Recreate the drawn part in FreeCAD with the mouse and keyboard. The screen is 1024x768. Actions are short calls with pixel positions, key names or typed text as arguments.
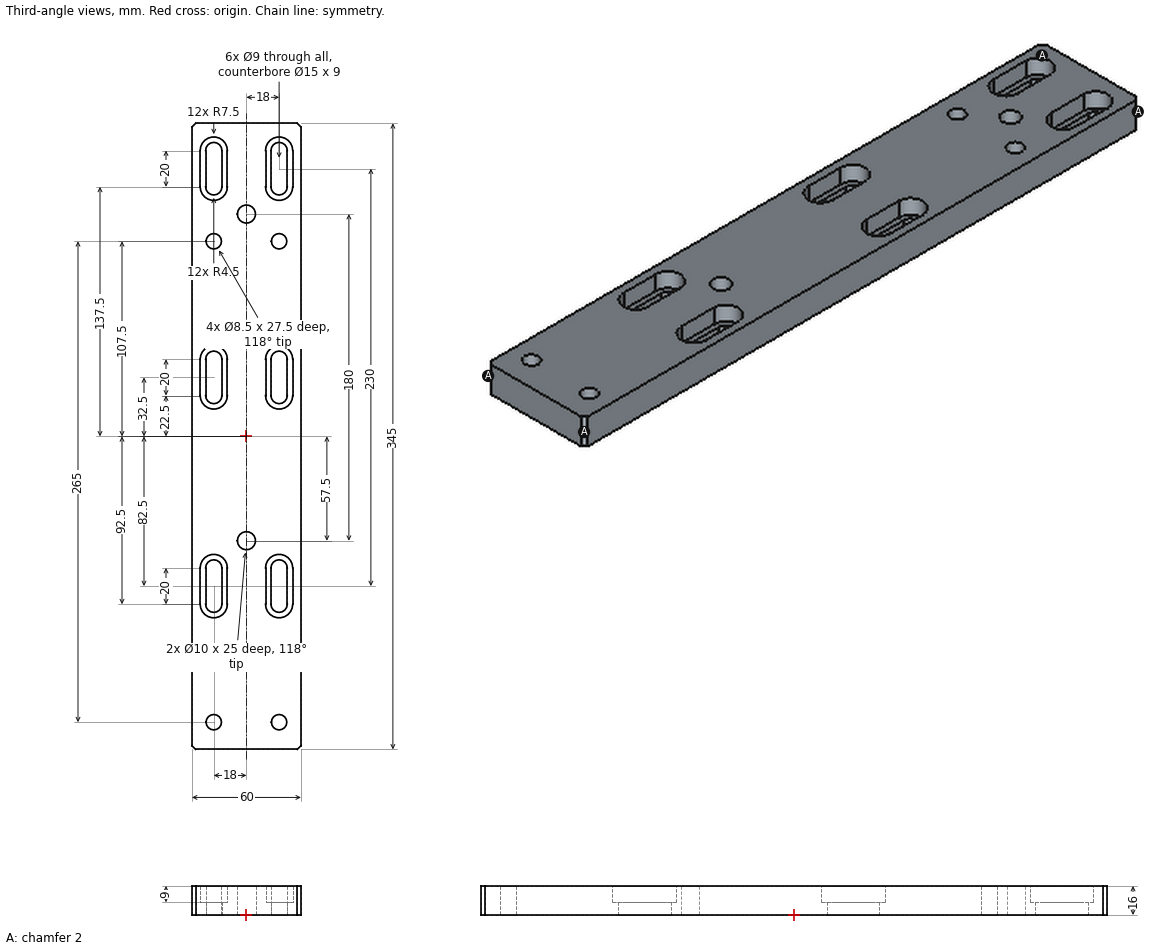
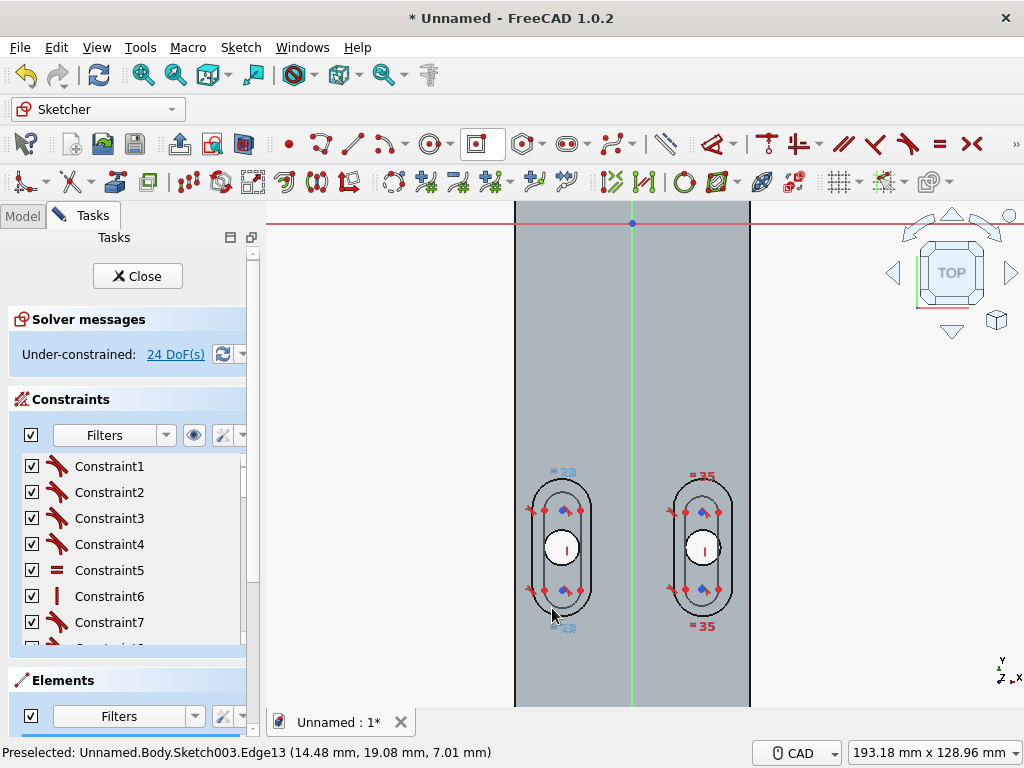
click(552, 605)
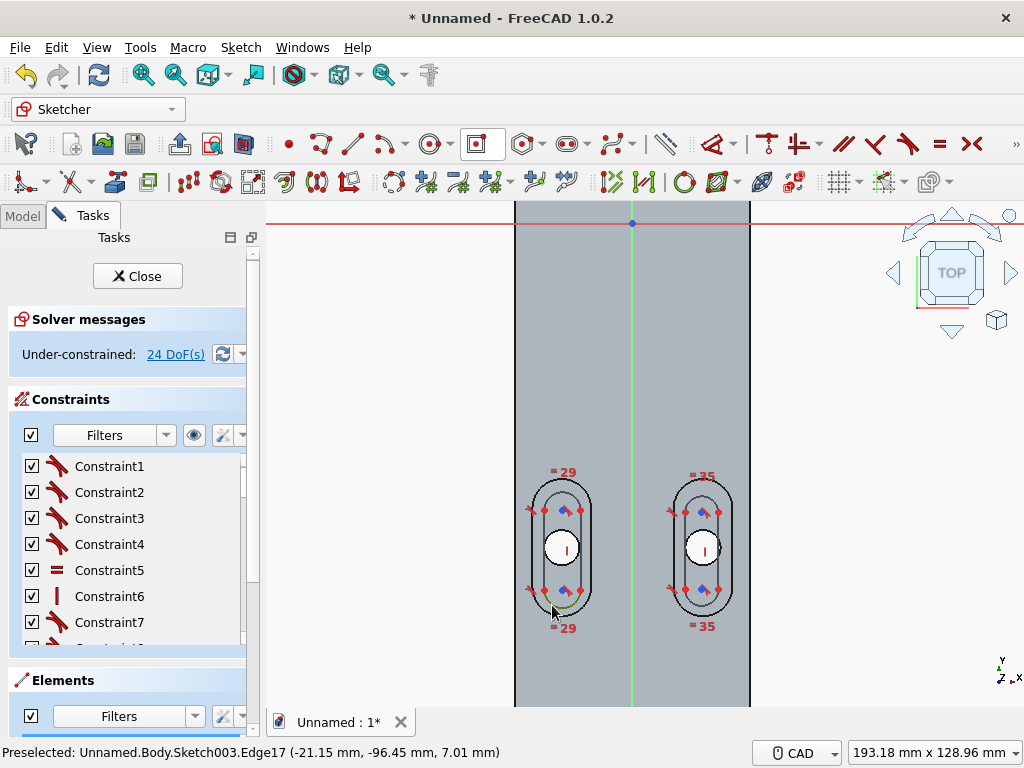
click(692, 603)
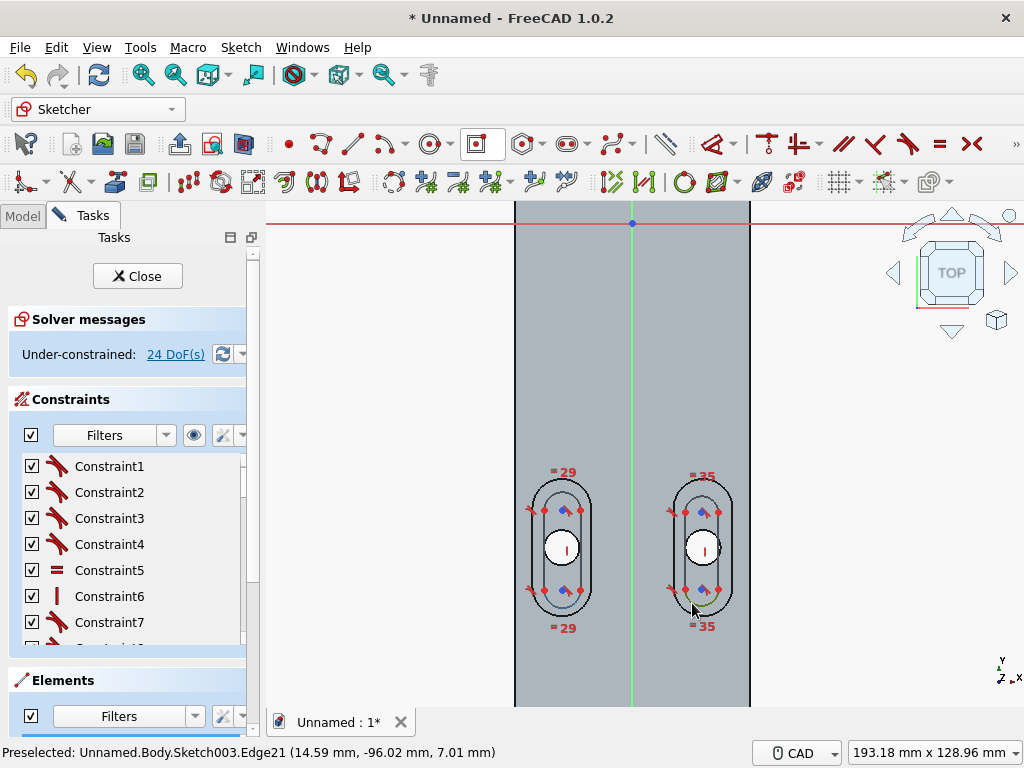
key(e)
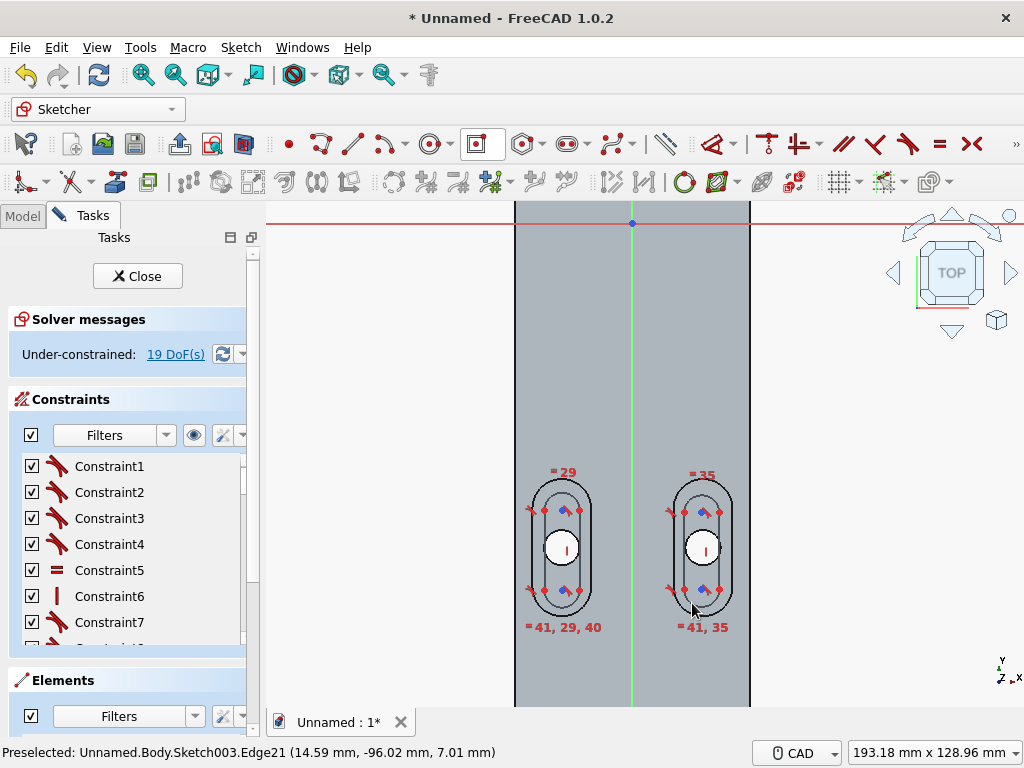
scroll(552, 608, down, 6)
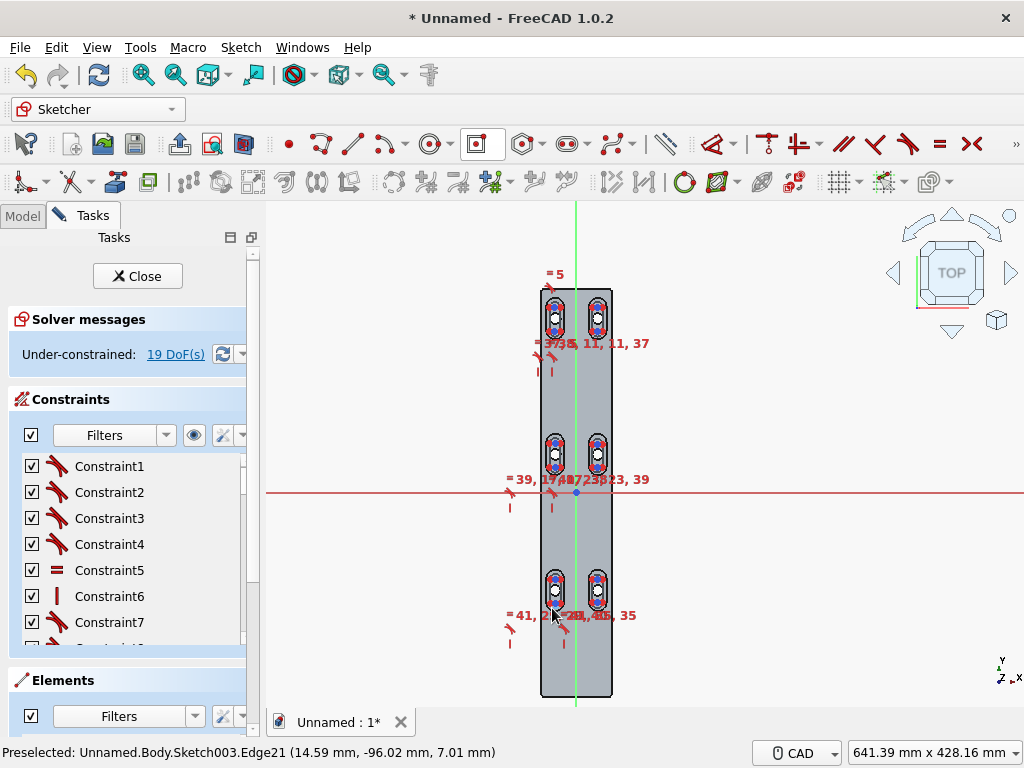
scroll(555, 331, up, 5)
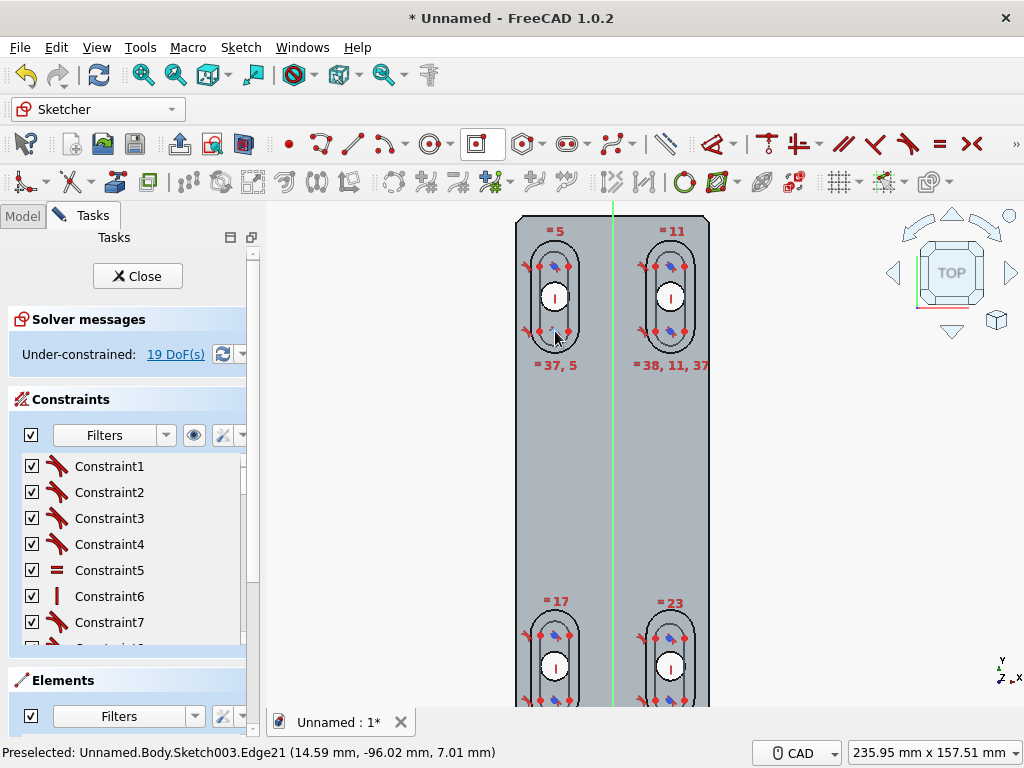
click(554, 331)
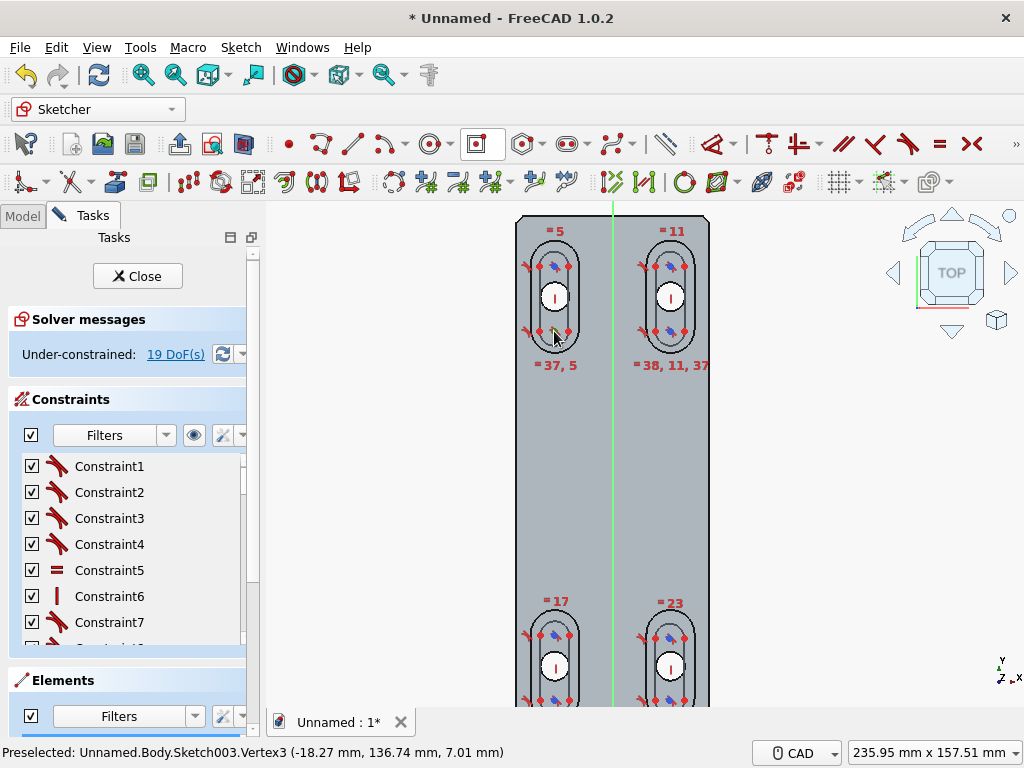
click(670, 331)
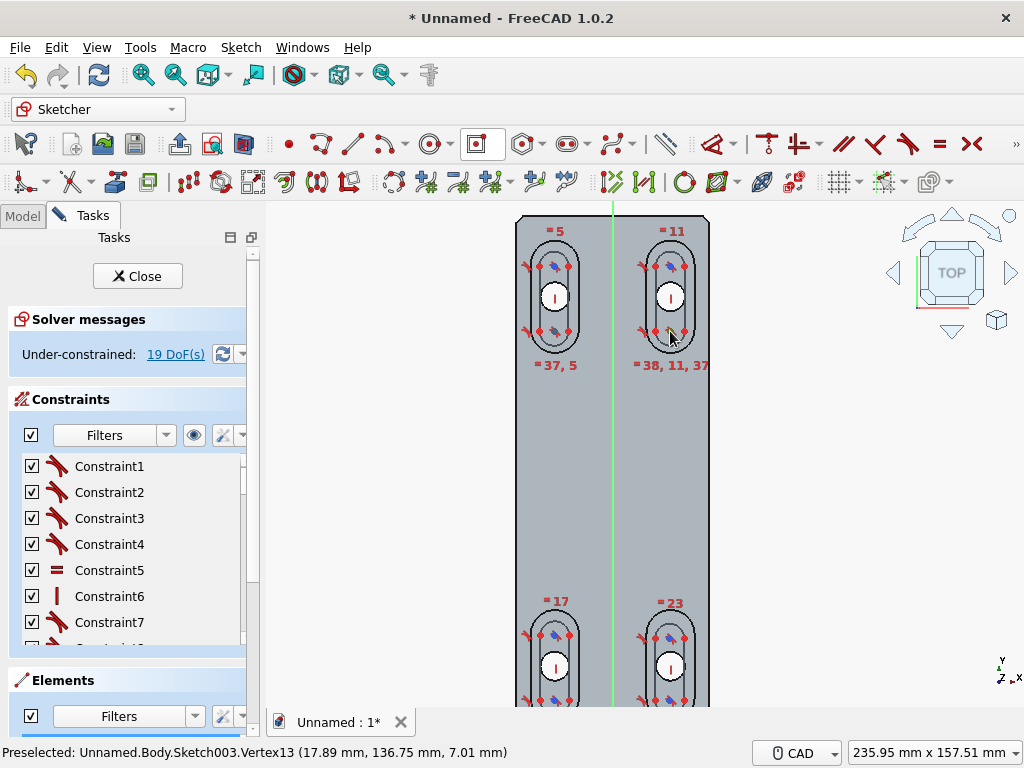
click(613, 647)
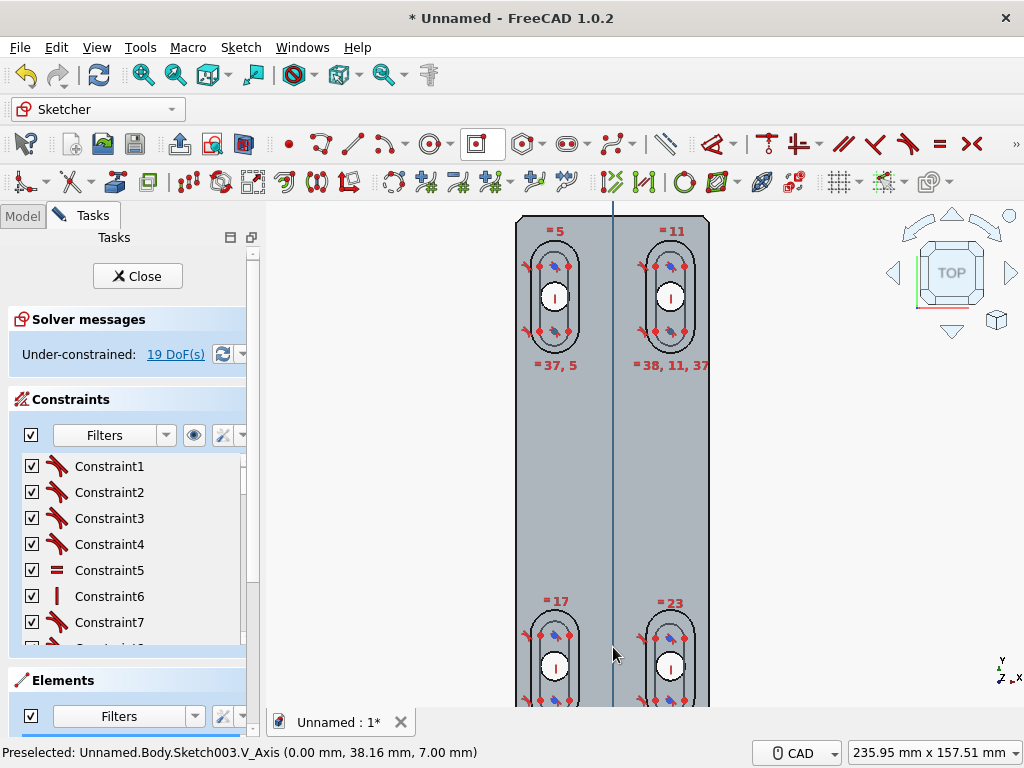
click(972, 144)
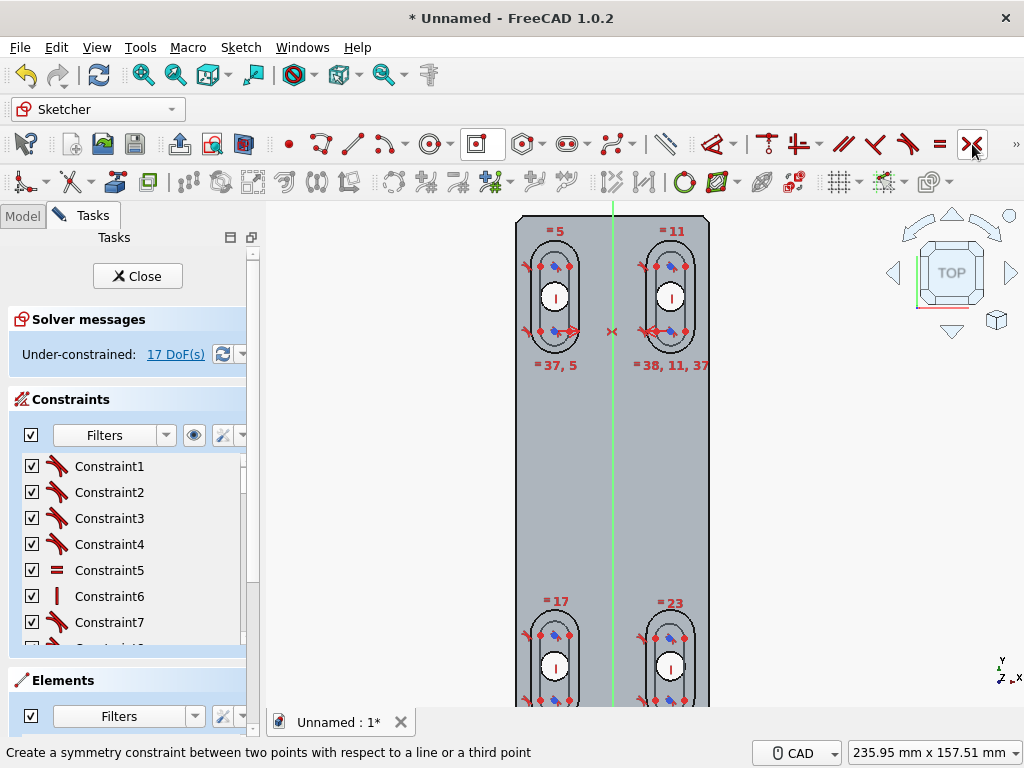
scroll(555, 331, down, 5)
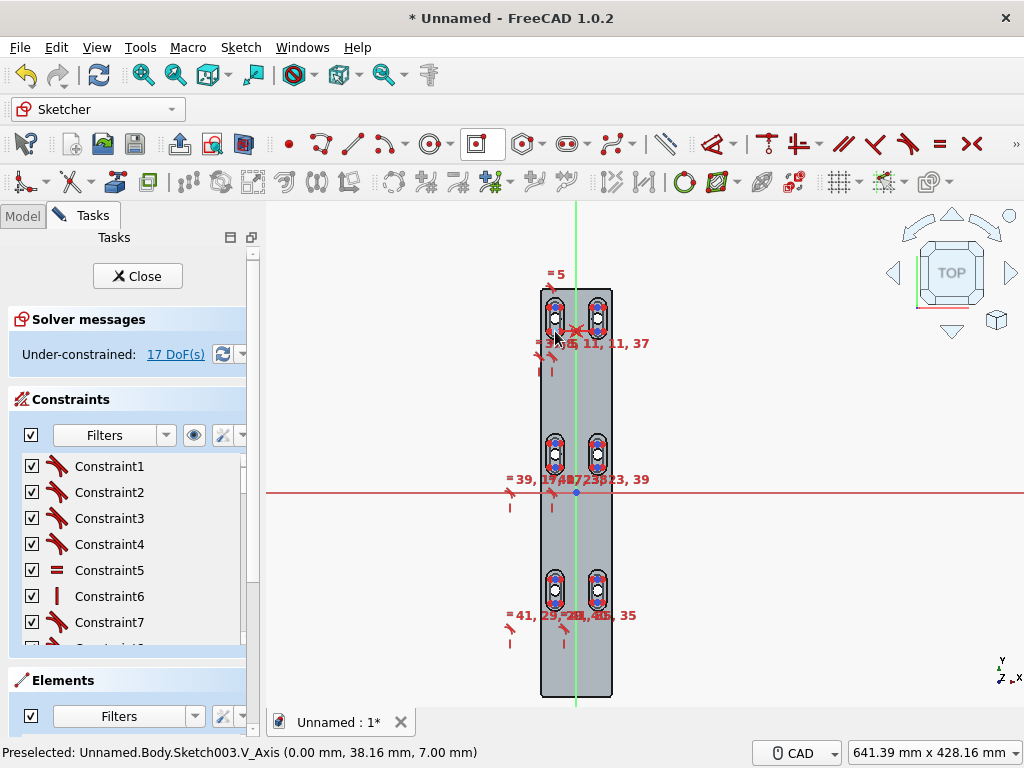
scroll(555, 467, up, 5)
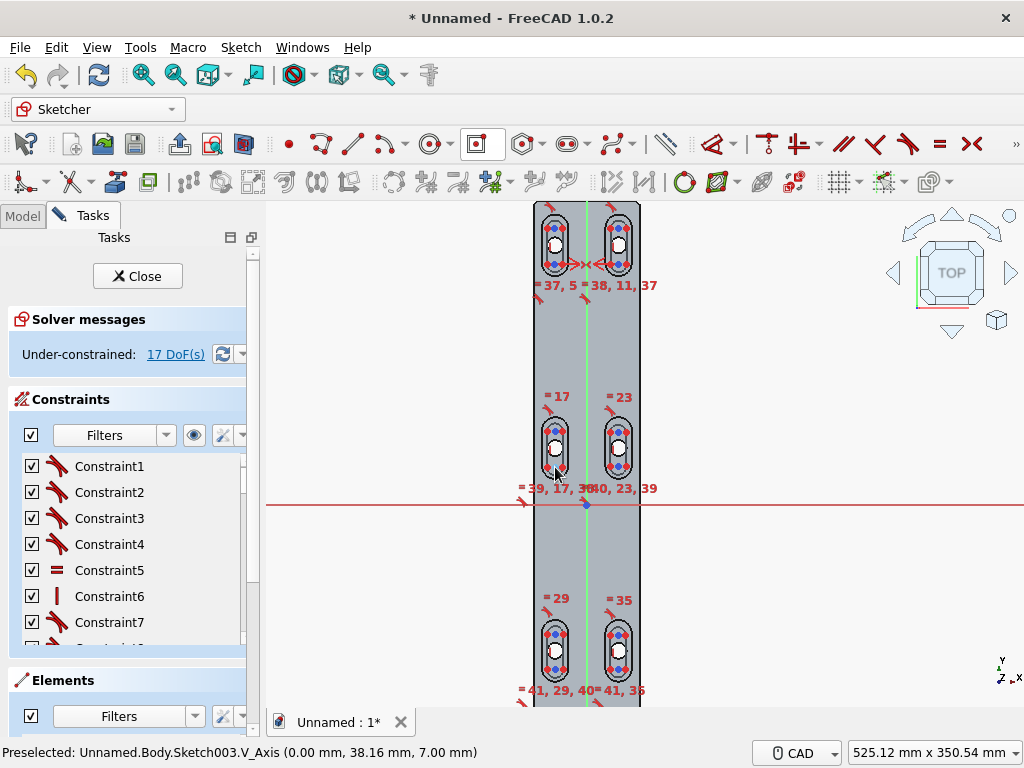
click(555, 467)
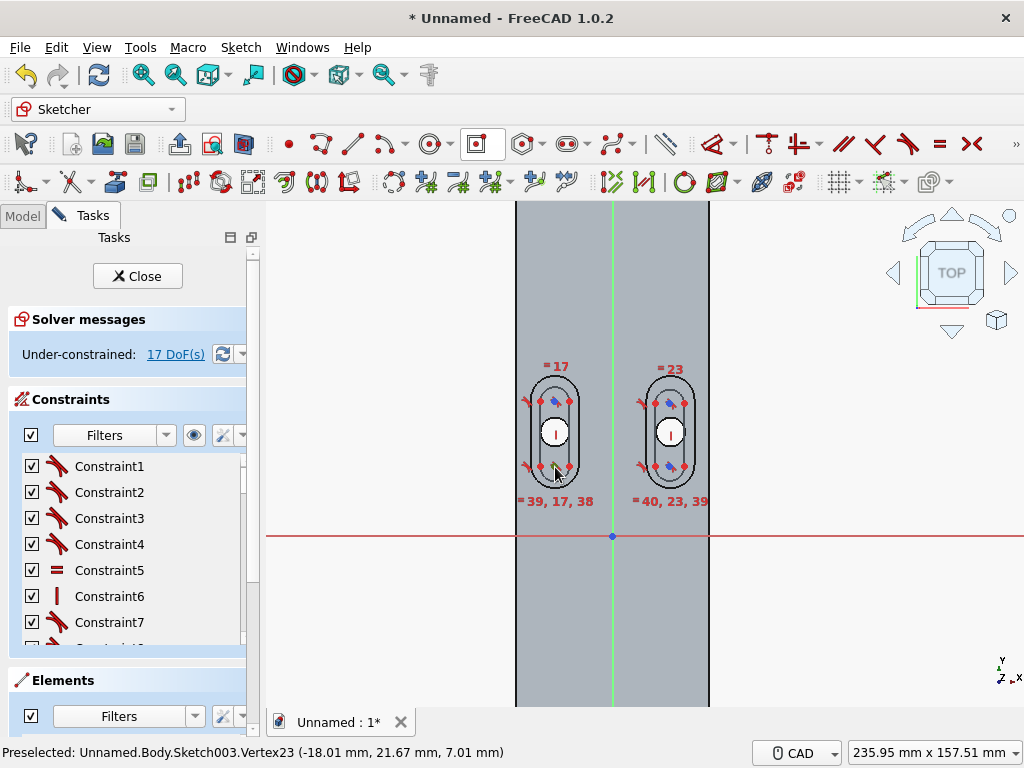
click(670, 467)